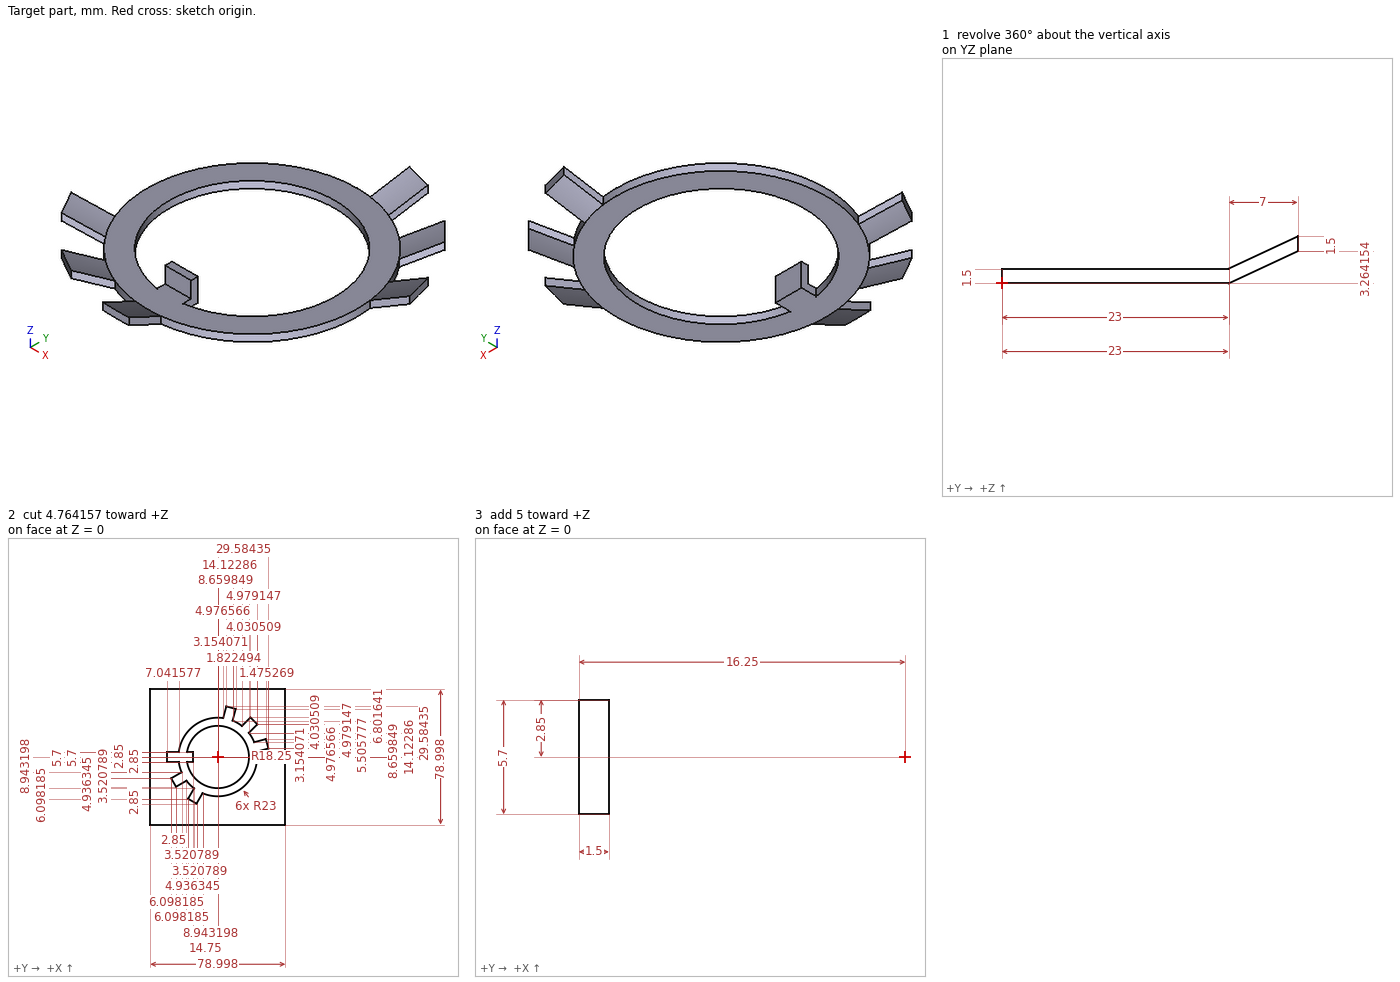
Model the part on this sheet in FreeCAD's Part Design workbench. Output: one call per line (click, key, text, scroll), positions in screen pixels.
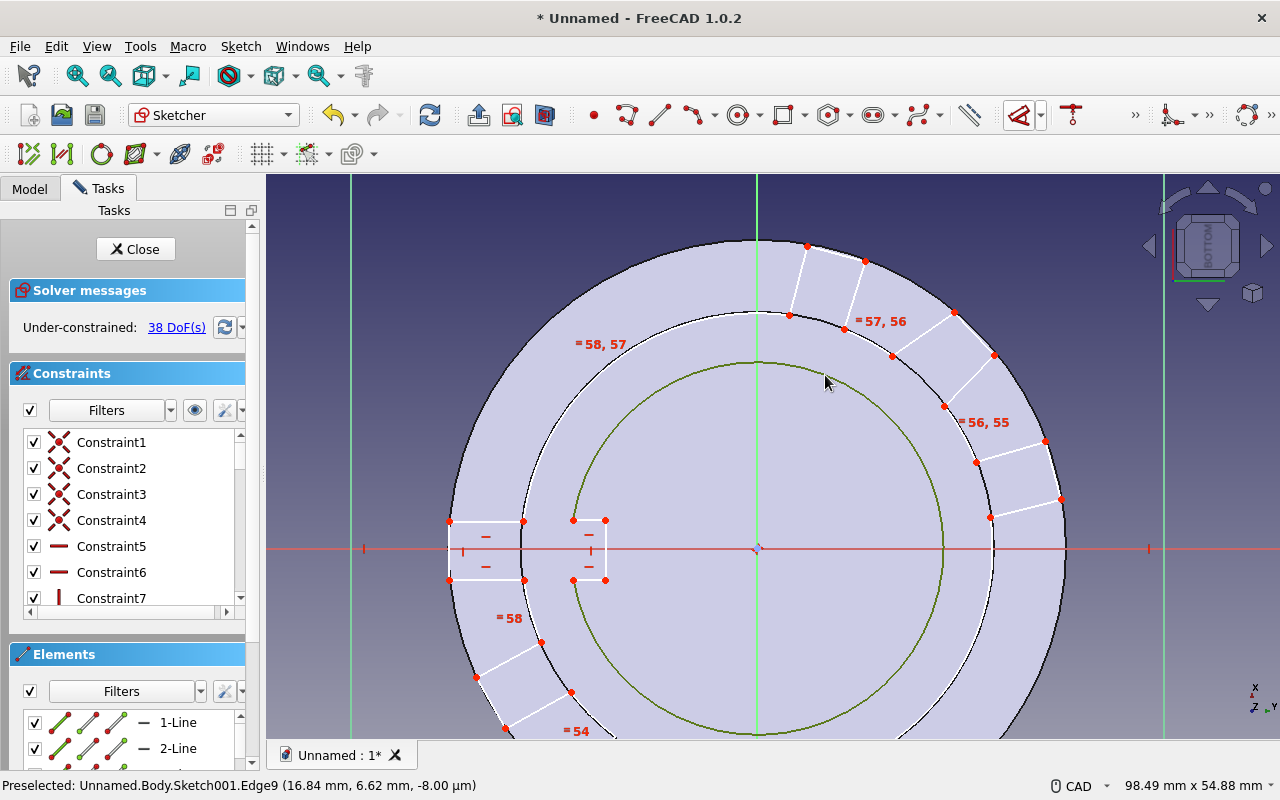
key(k)
key(r)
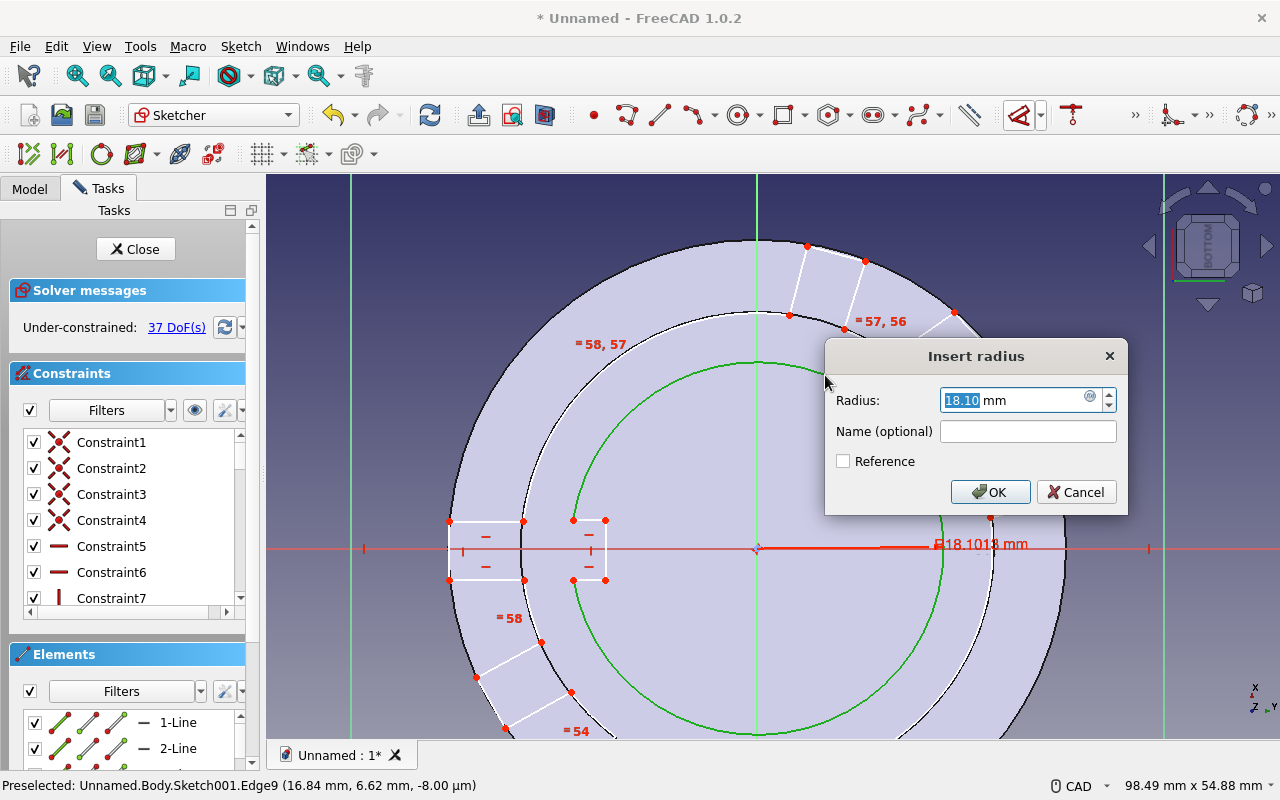
text(18.25)
key(Return)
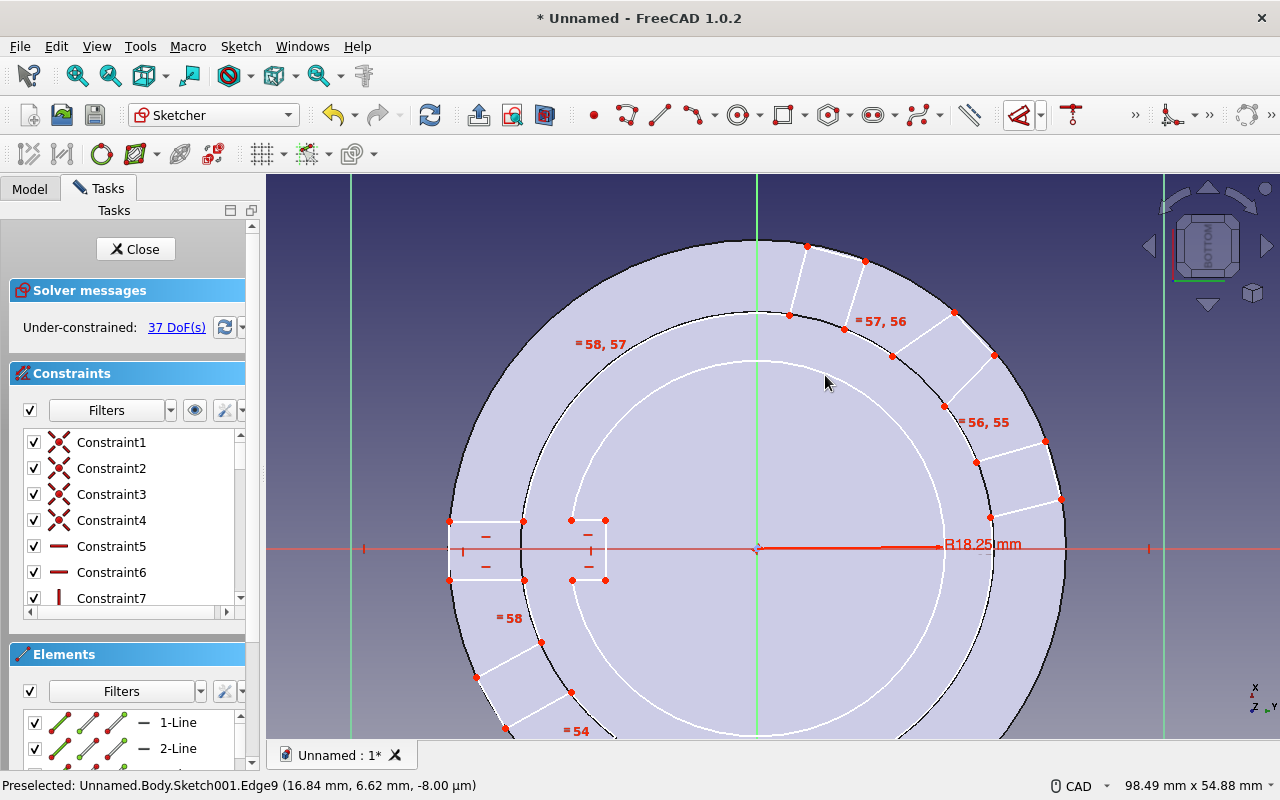
click(583, 707)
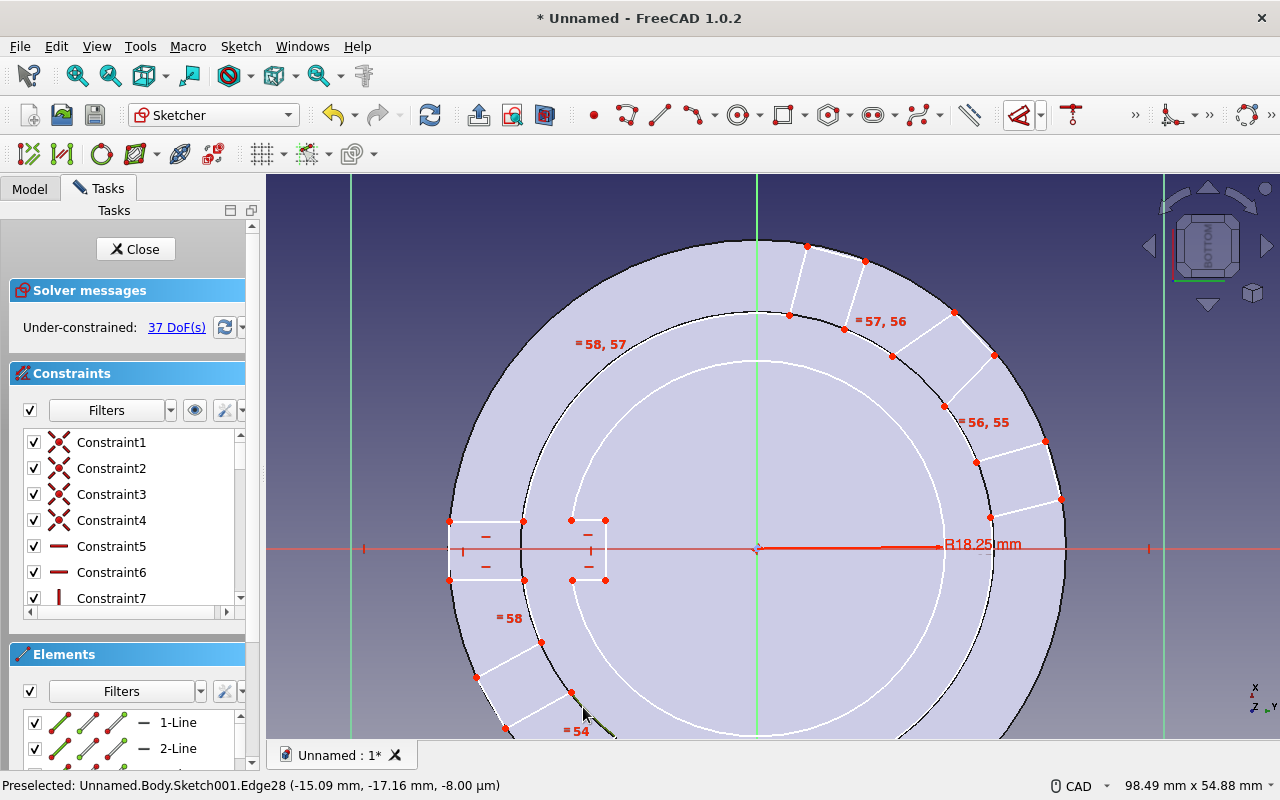
key(k)
key(r)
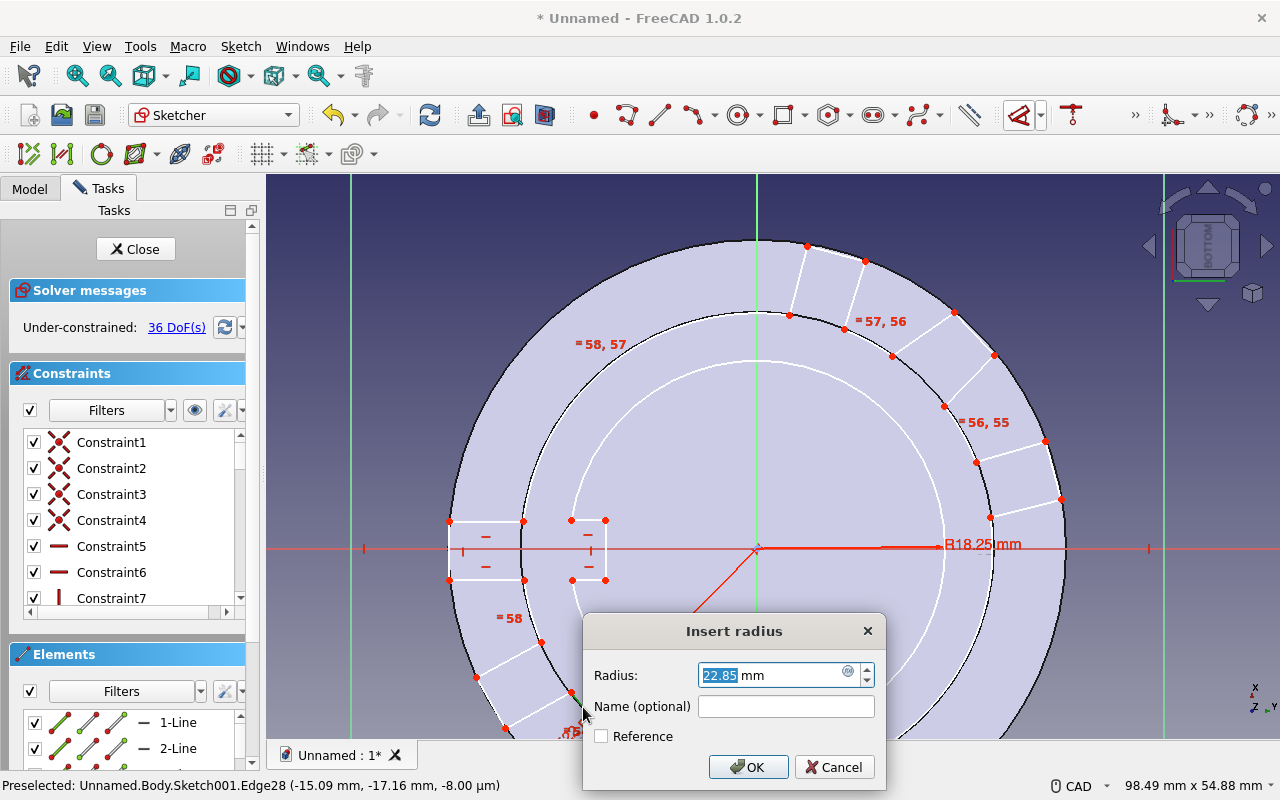
text(23)
key(Return)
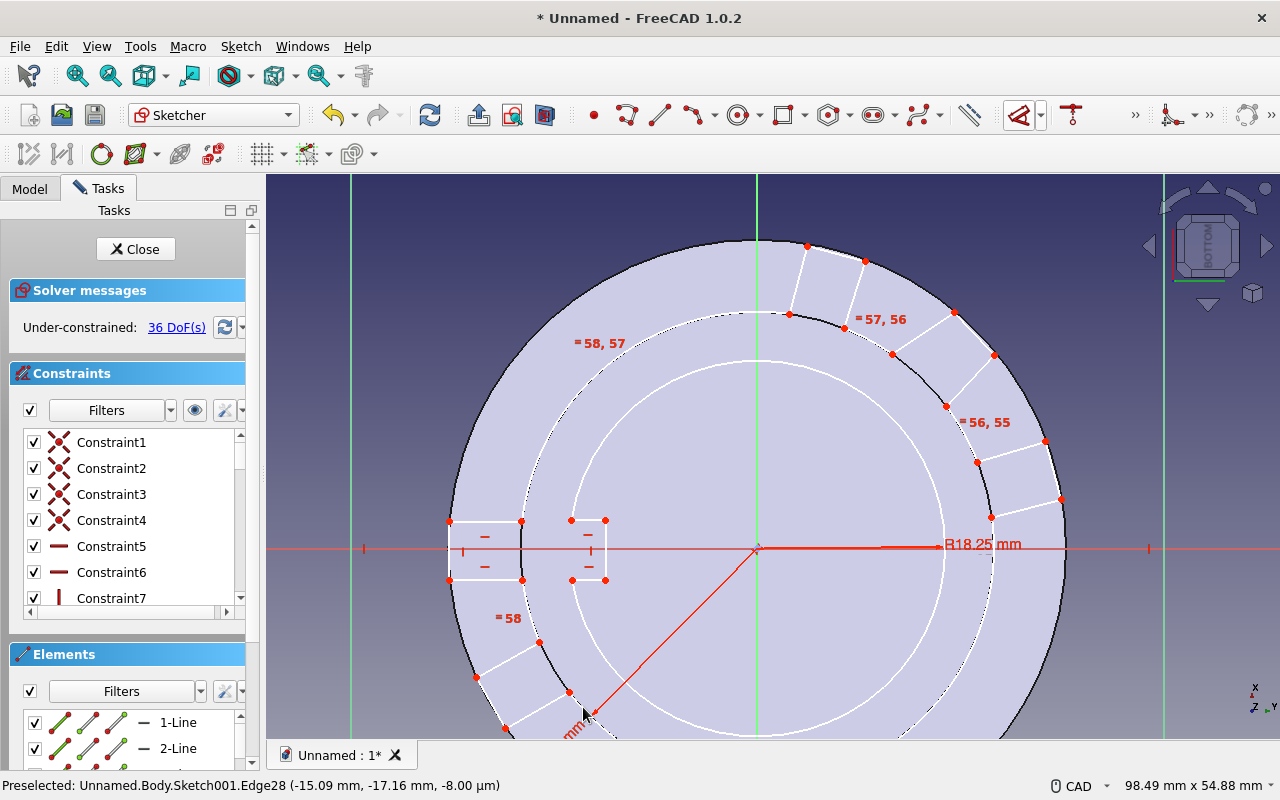
click(606, 562)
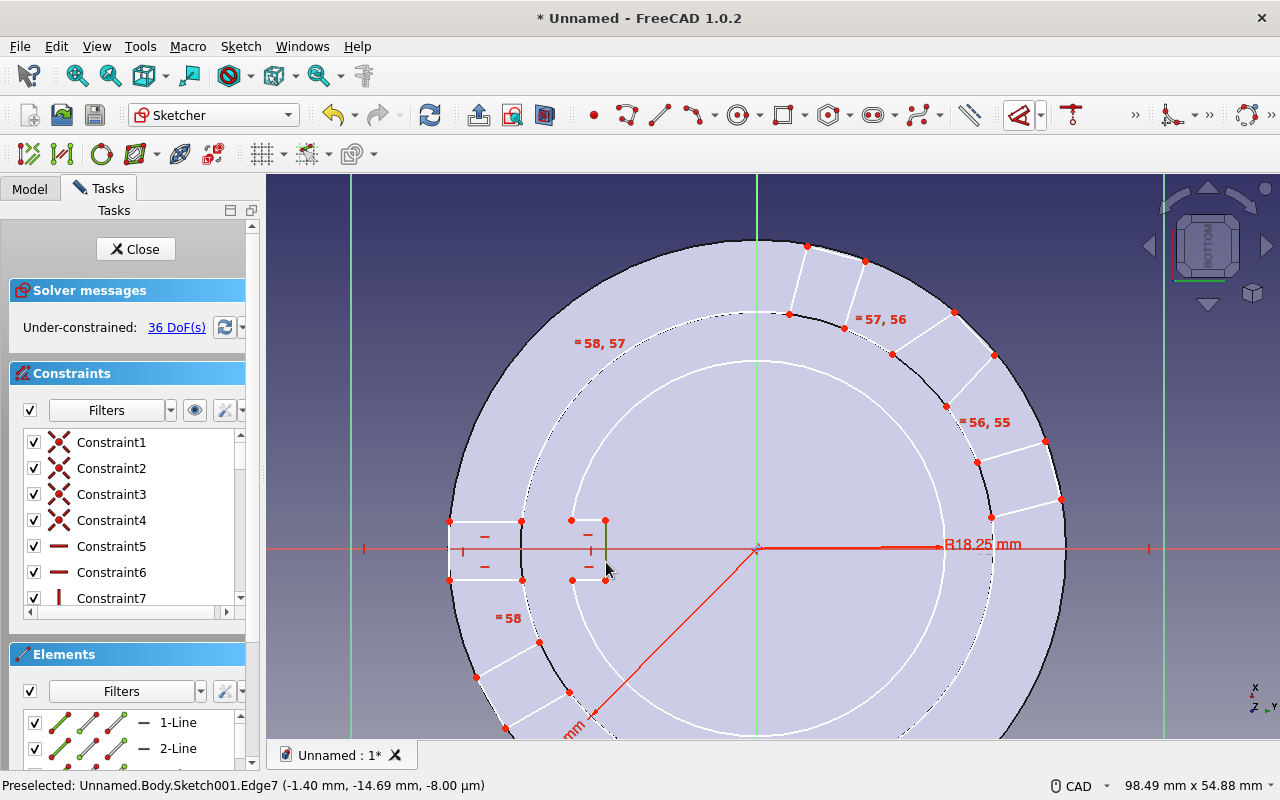
click(1040, 116)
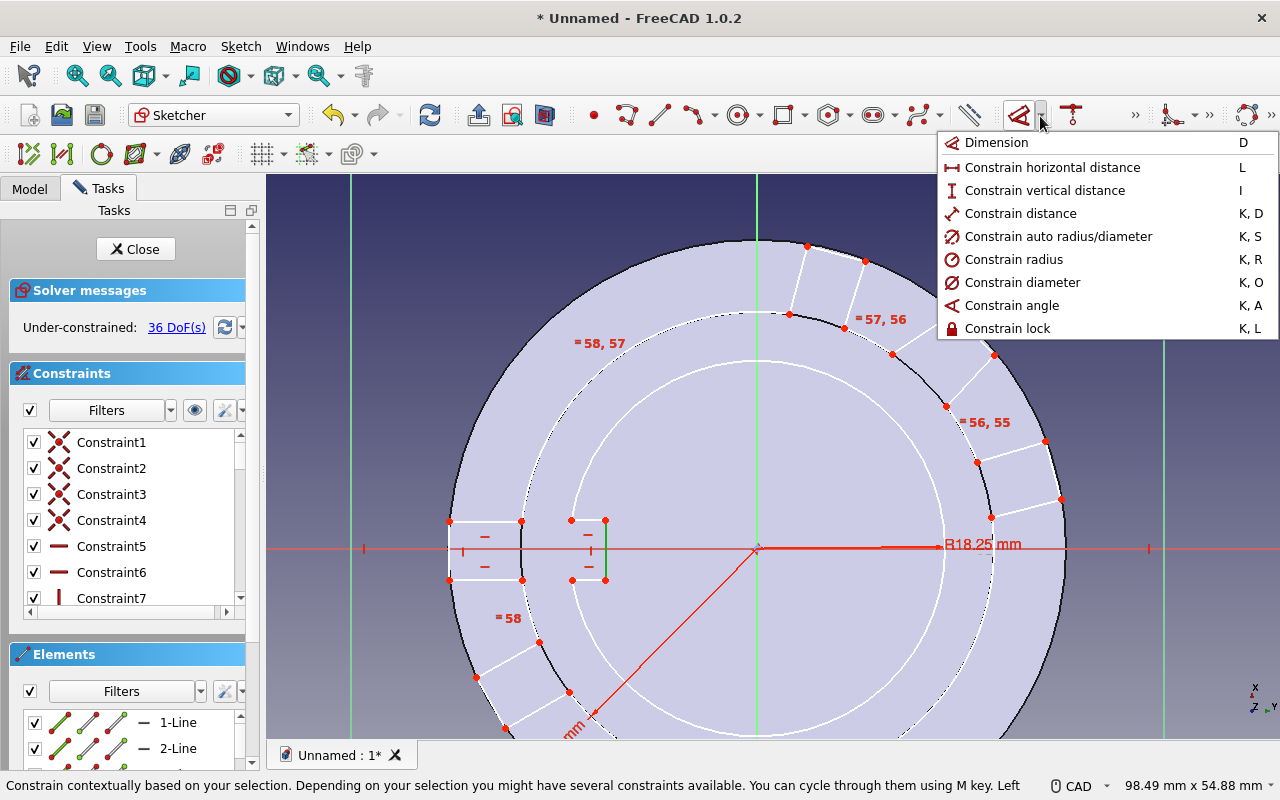
click(1108, 190)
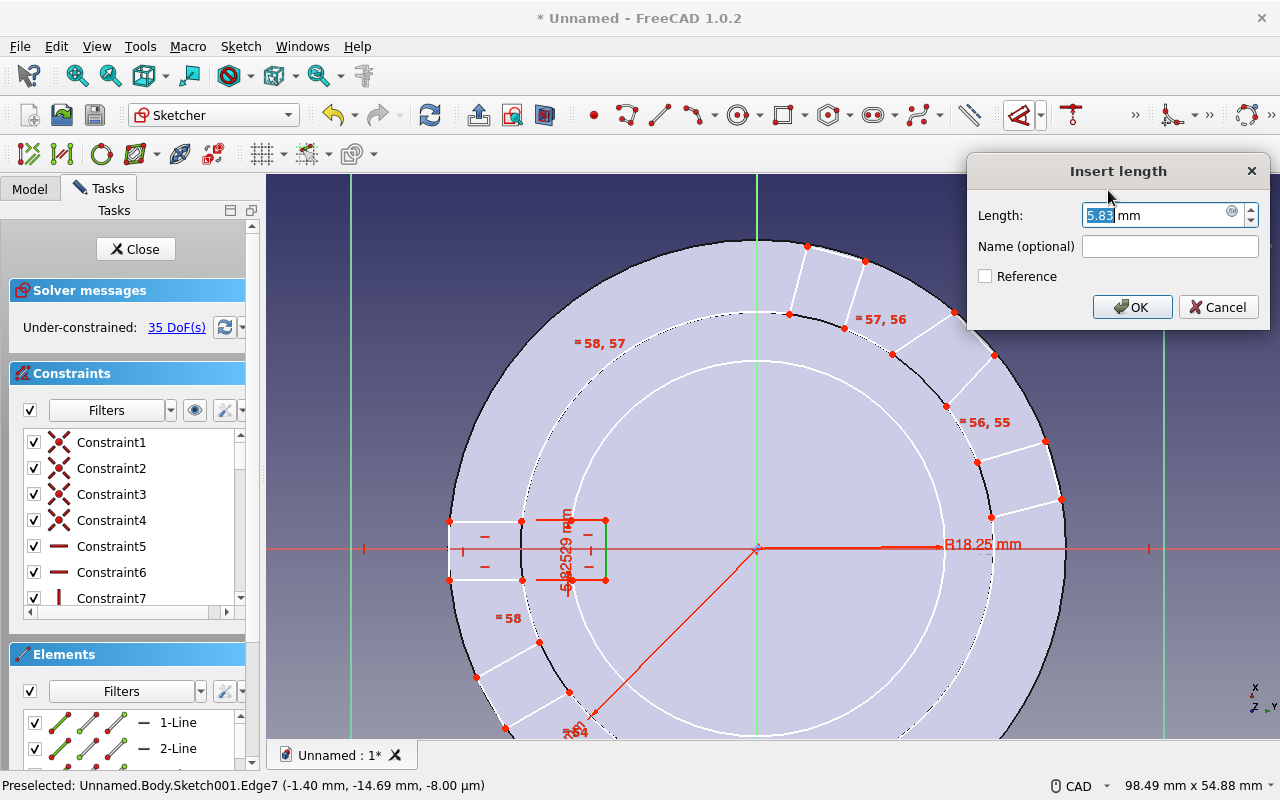
text(5.7)
key(Return)